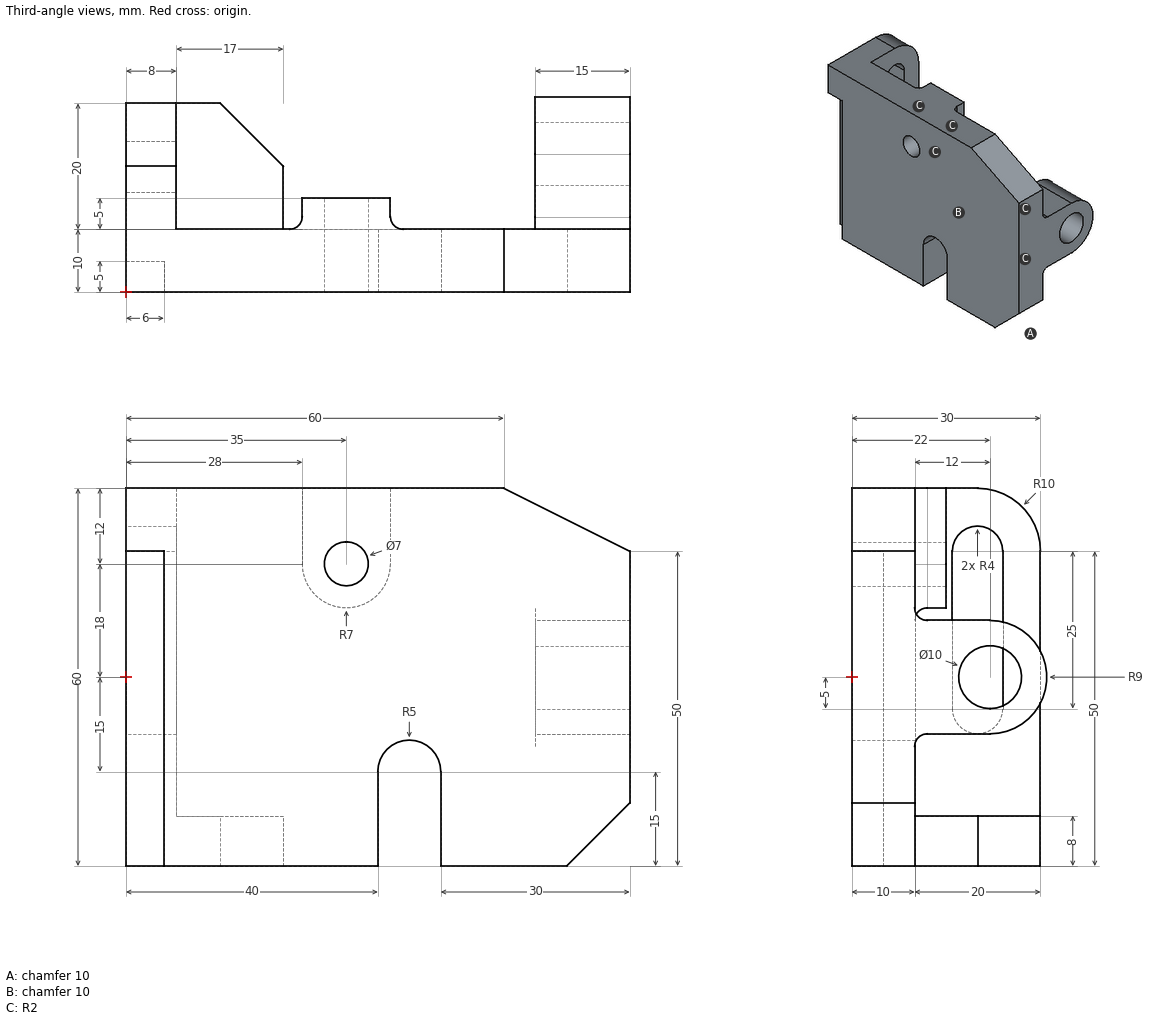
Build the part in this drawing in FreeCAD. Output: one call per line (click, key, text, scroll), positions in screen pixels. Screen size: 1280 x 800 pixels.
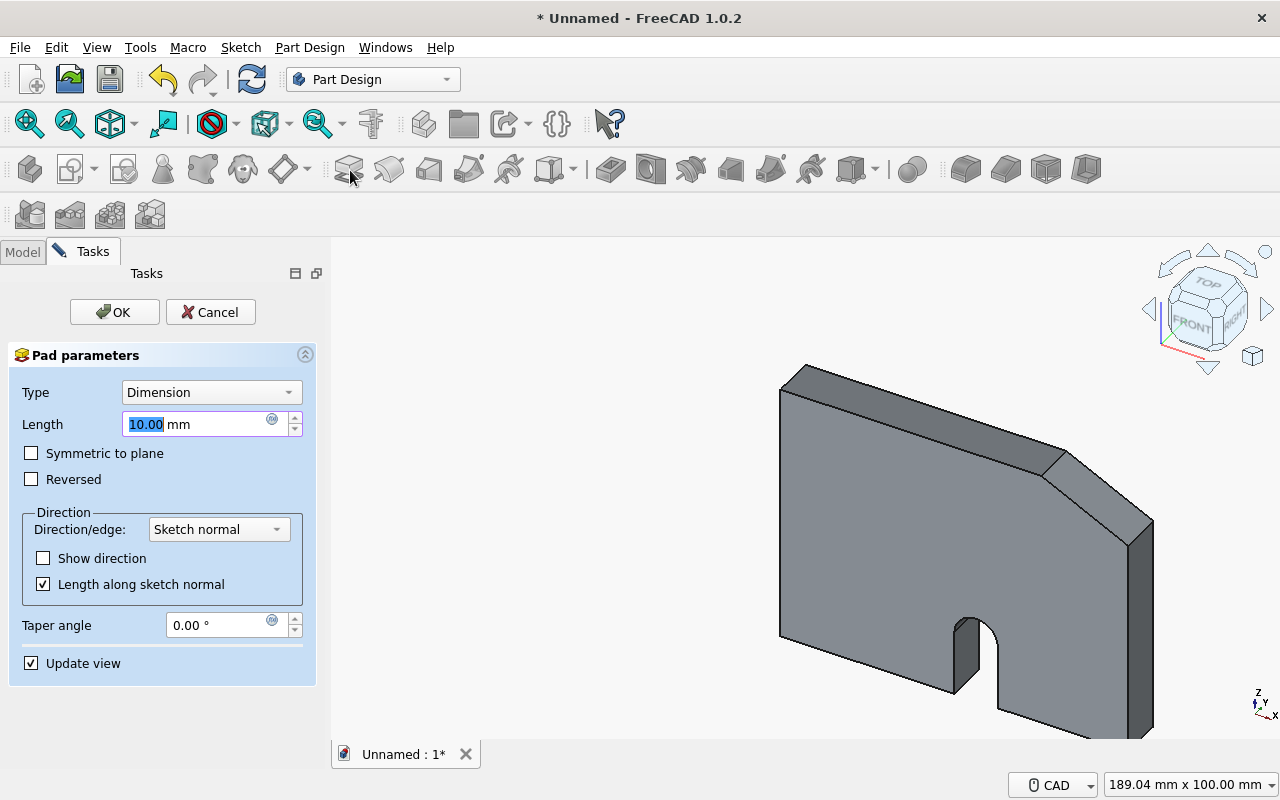
text(10)
key(Tab)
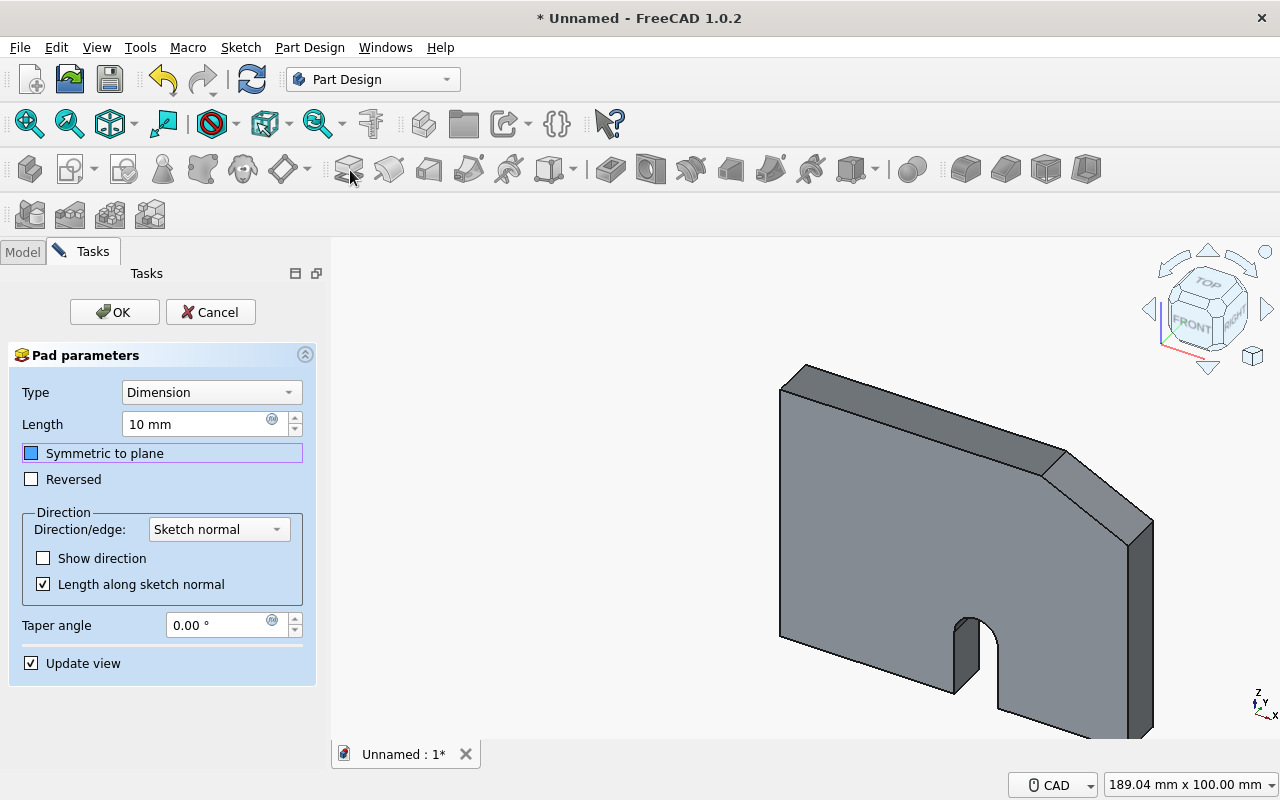
click(30, 479)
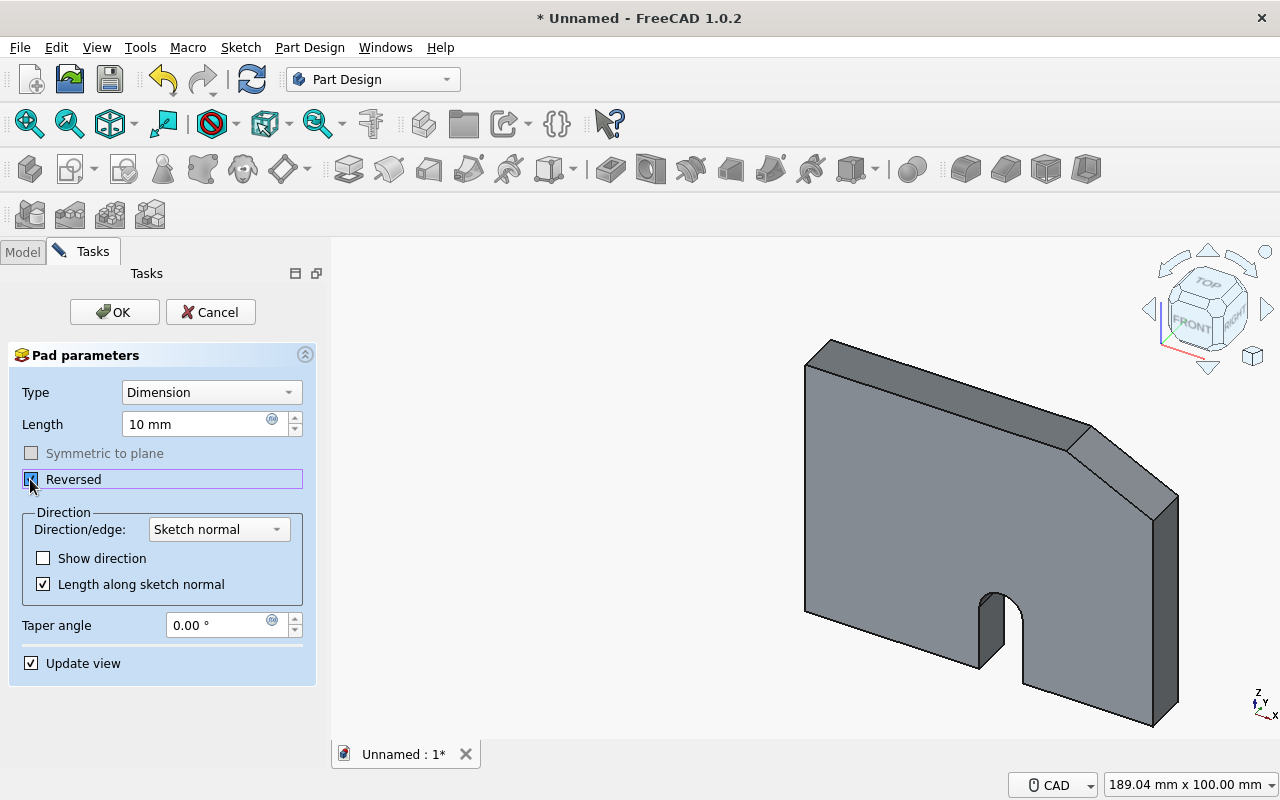
click(115, 312)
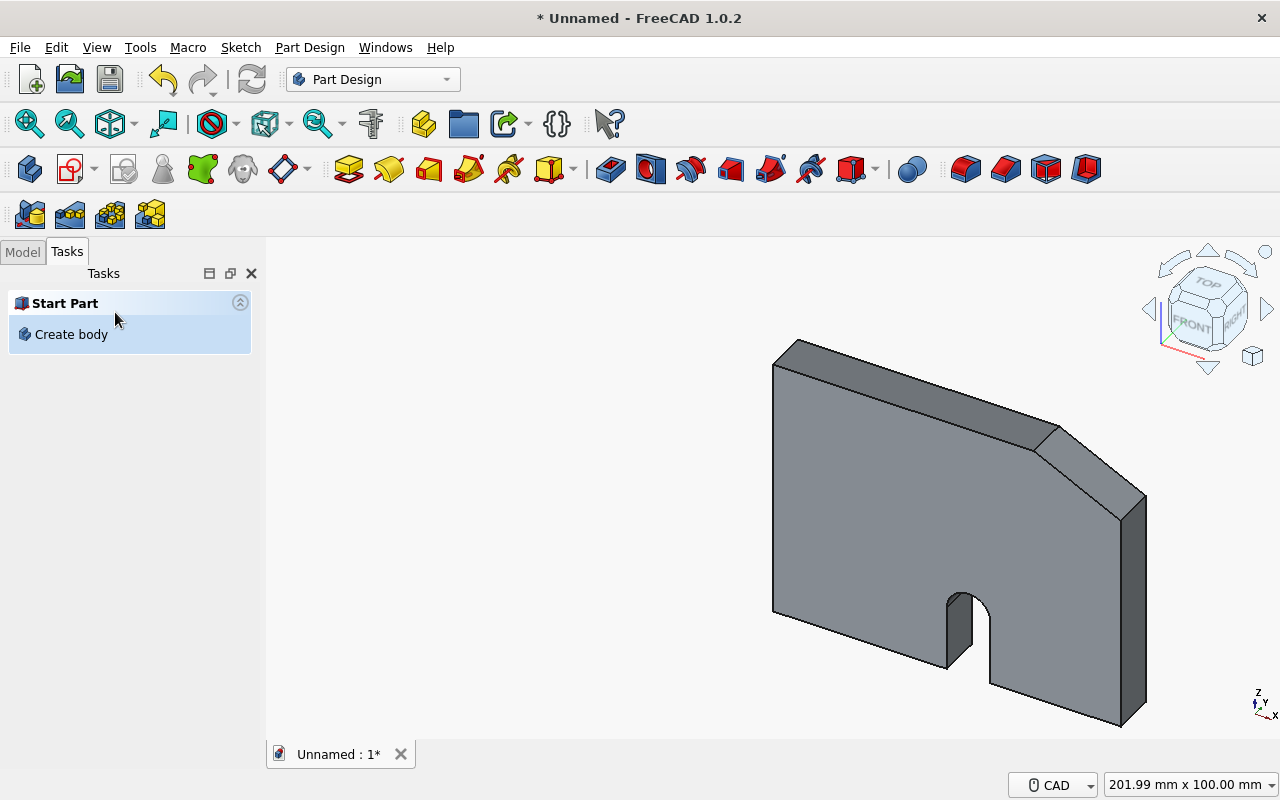
key(0)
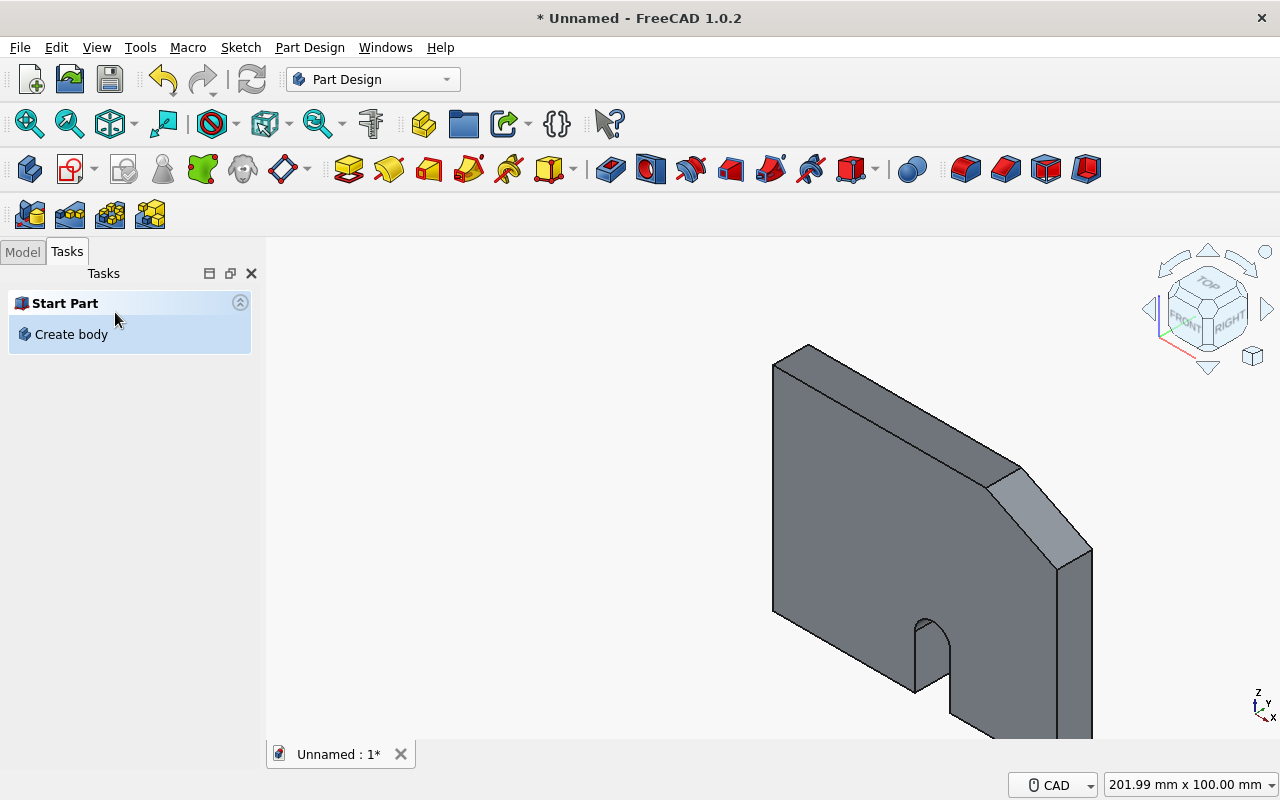
click(30, 124)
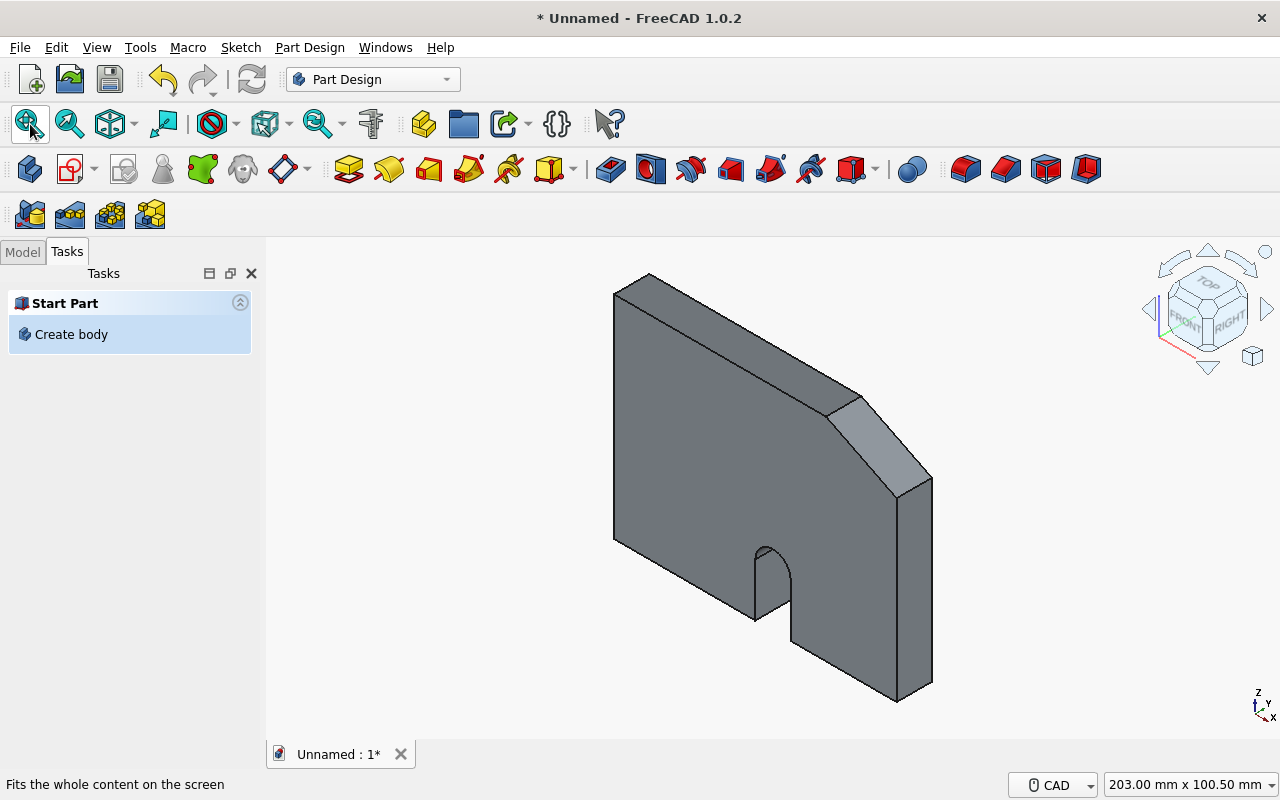
key(2)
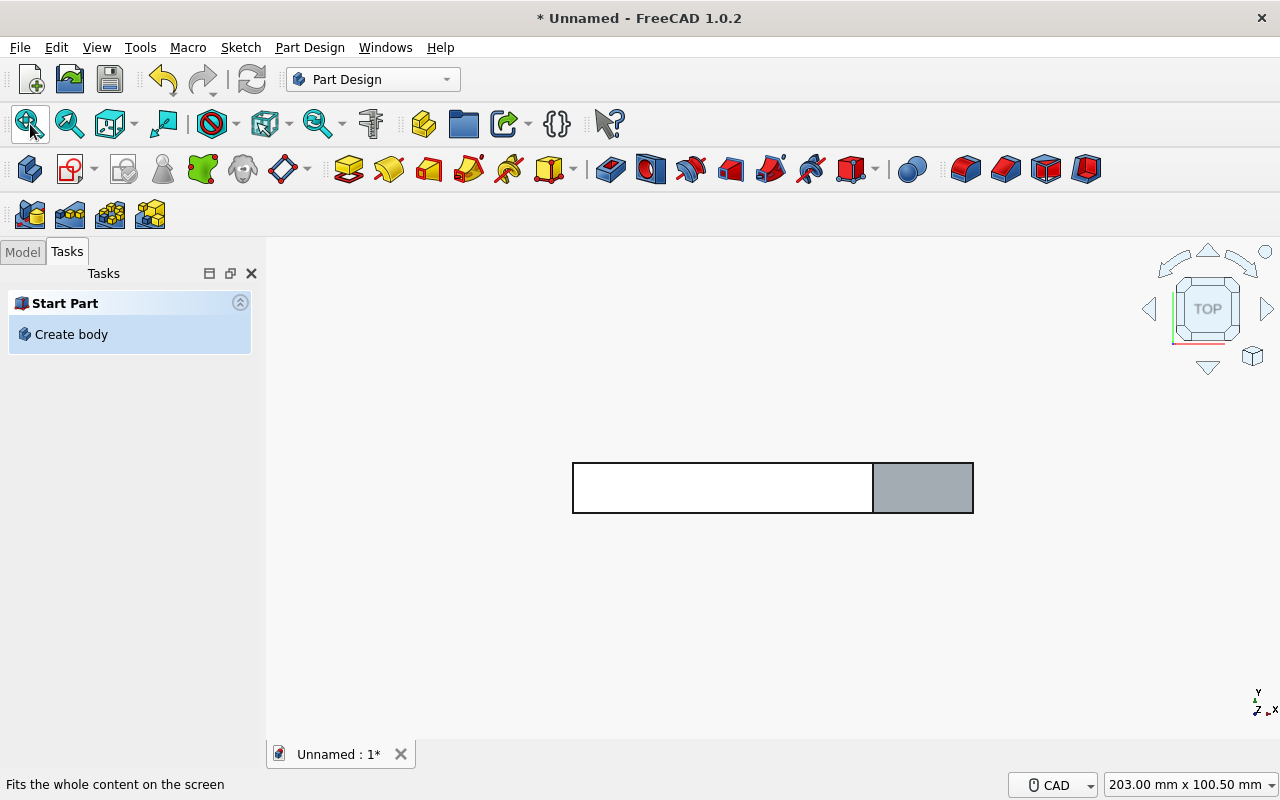
key(v)
key(f)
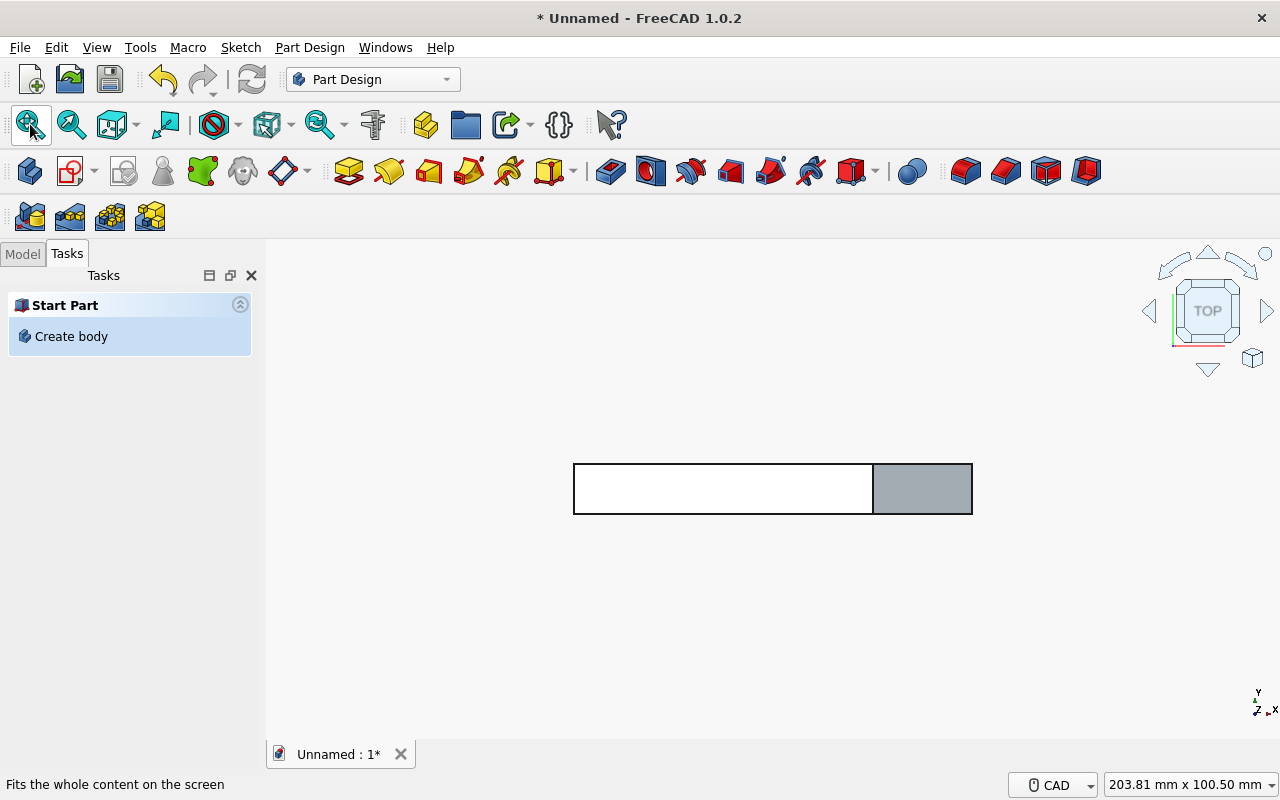
key(1)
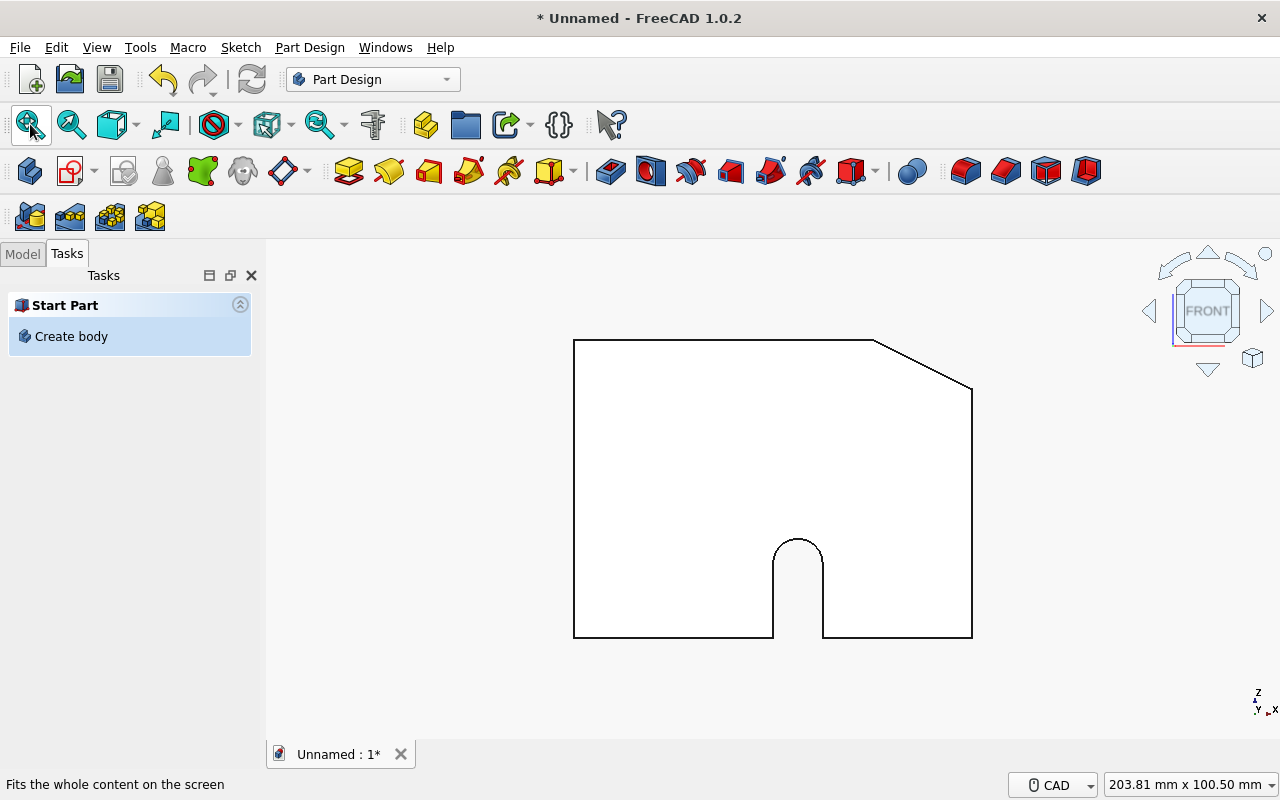
key(3)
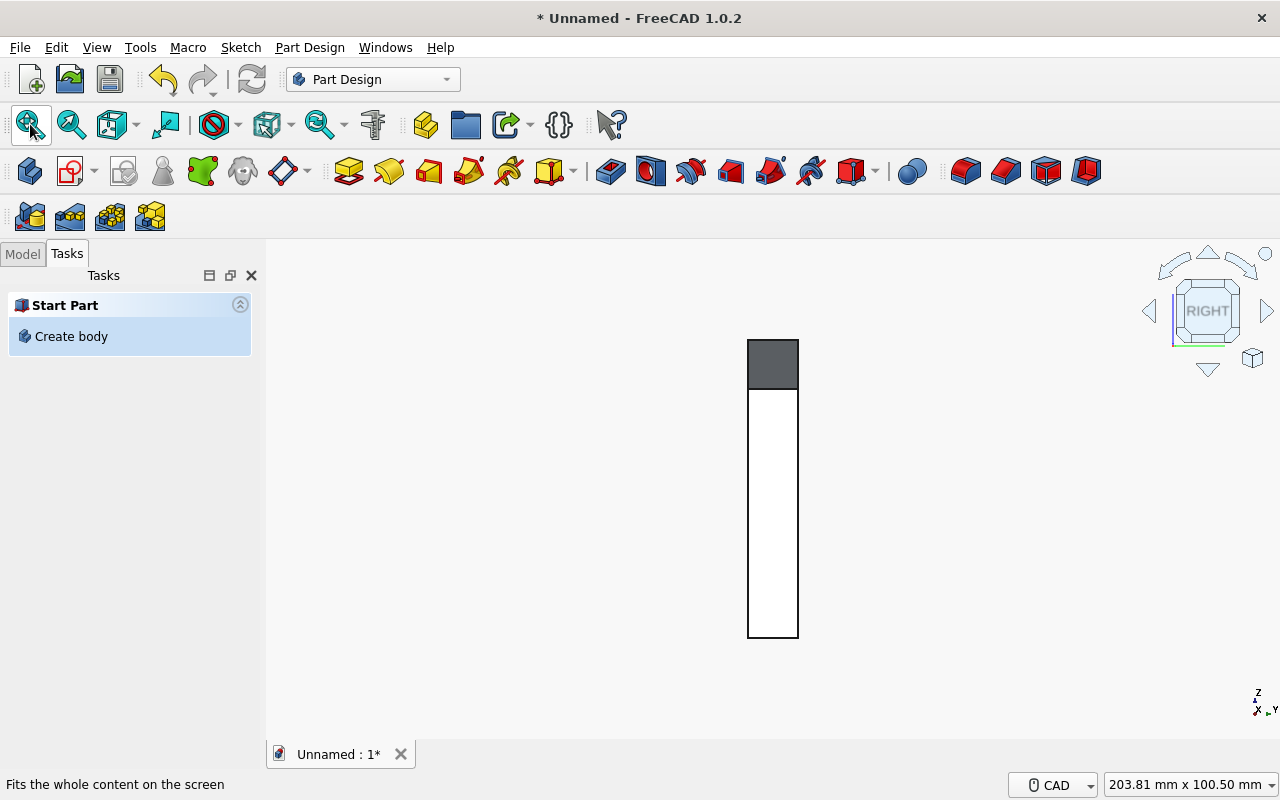
click(773, 637)